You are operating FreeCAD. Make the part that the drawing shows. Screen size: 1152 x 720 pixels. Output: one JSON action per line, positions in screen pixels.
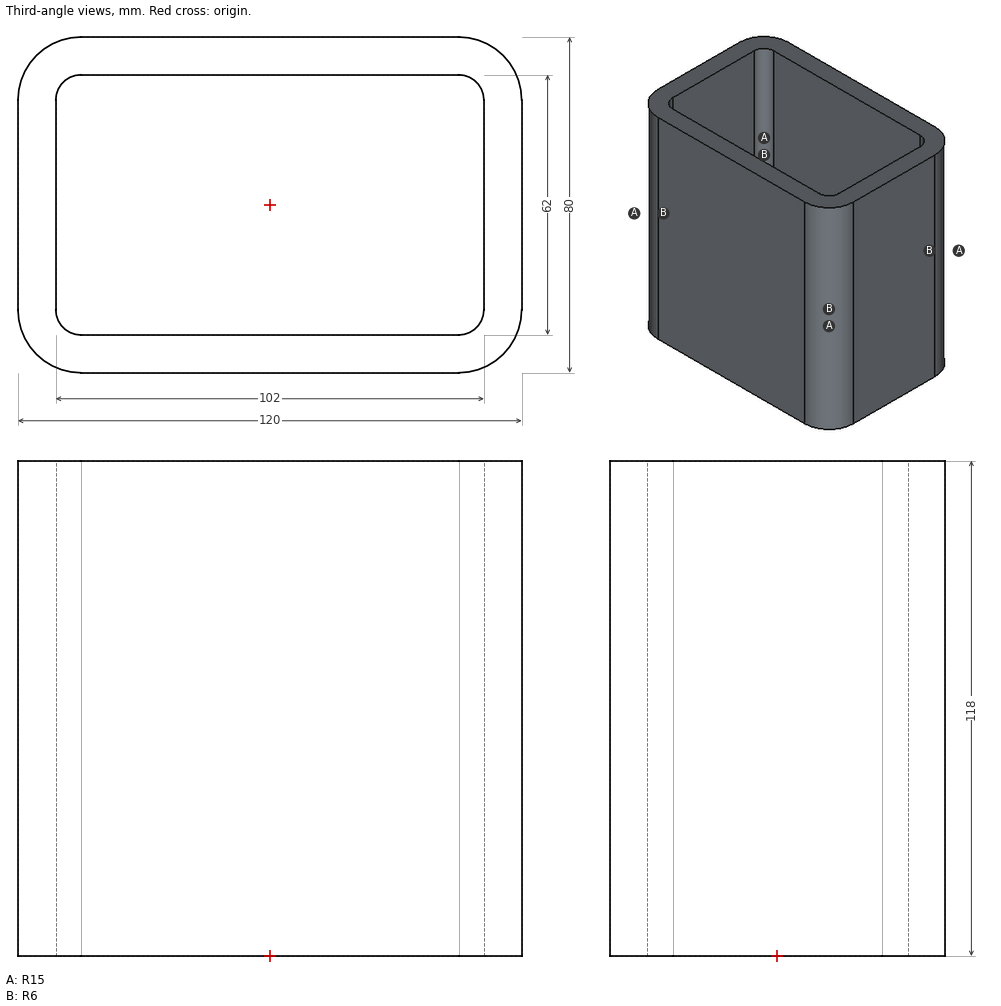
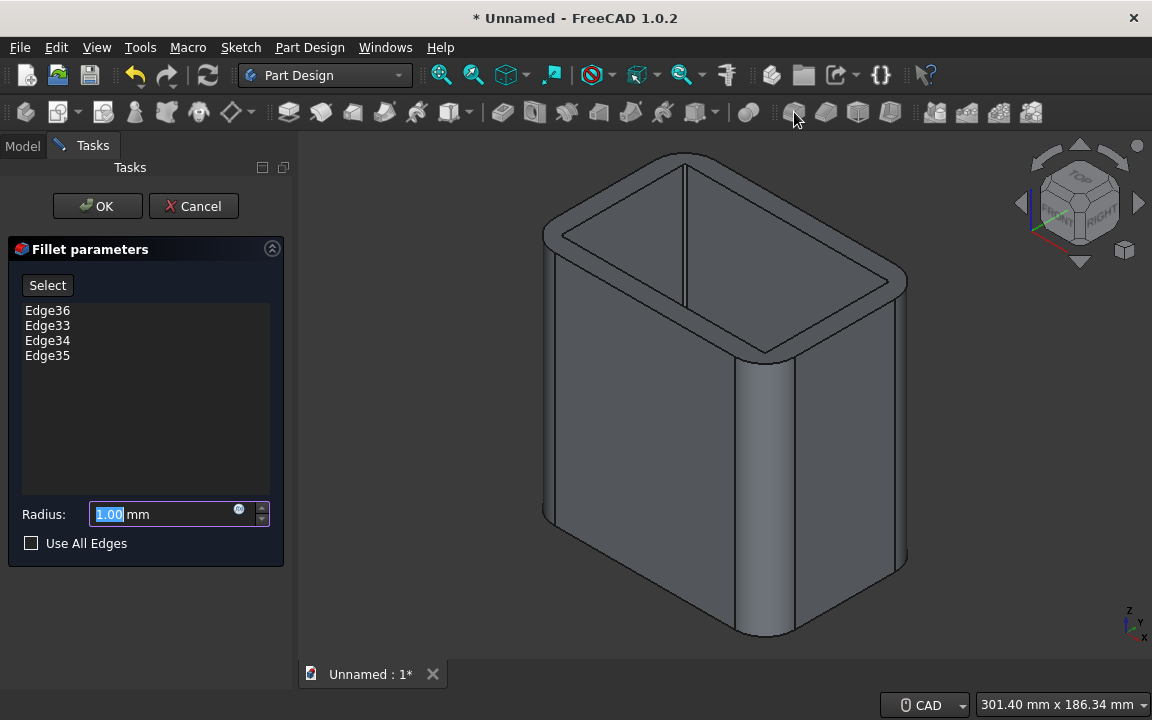
{"action": "type", "text": "6"}
{"action": "key", "text": "Tab"}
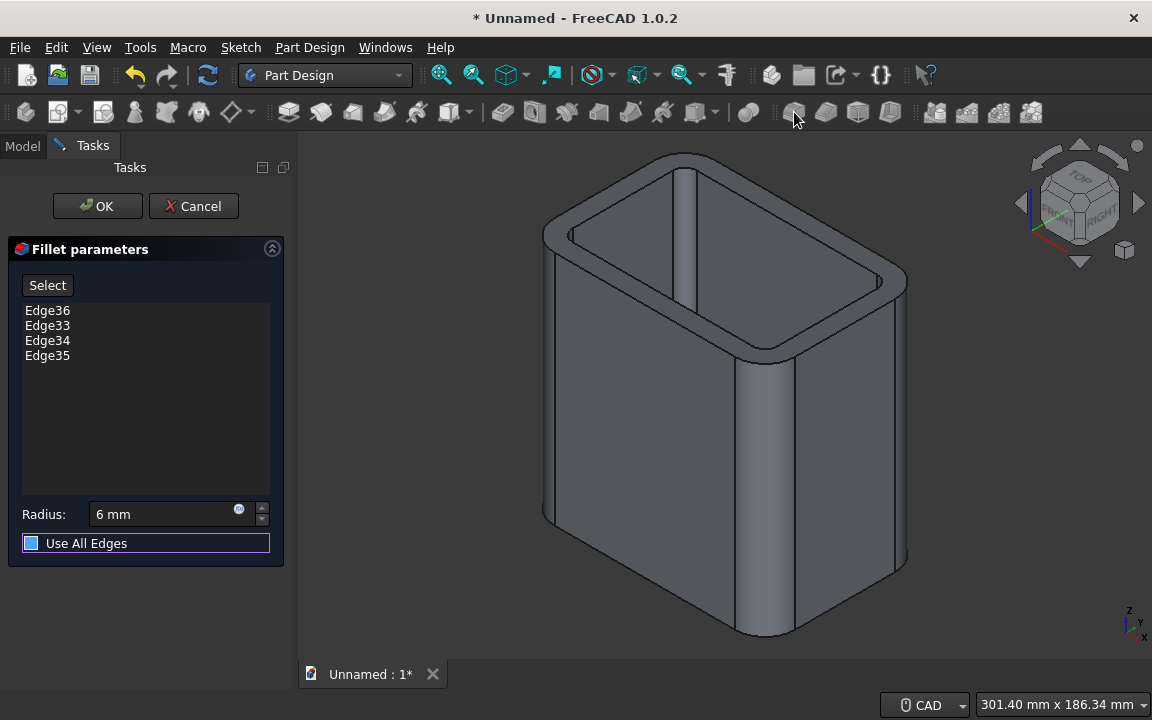
{"action": "left_click", "coordinate": [98, 206]}